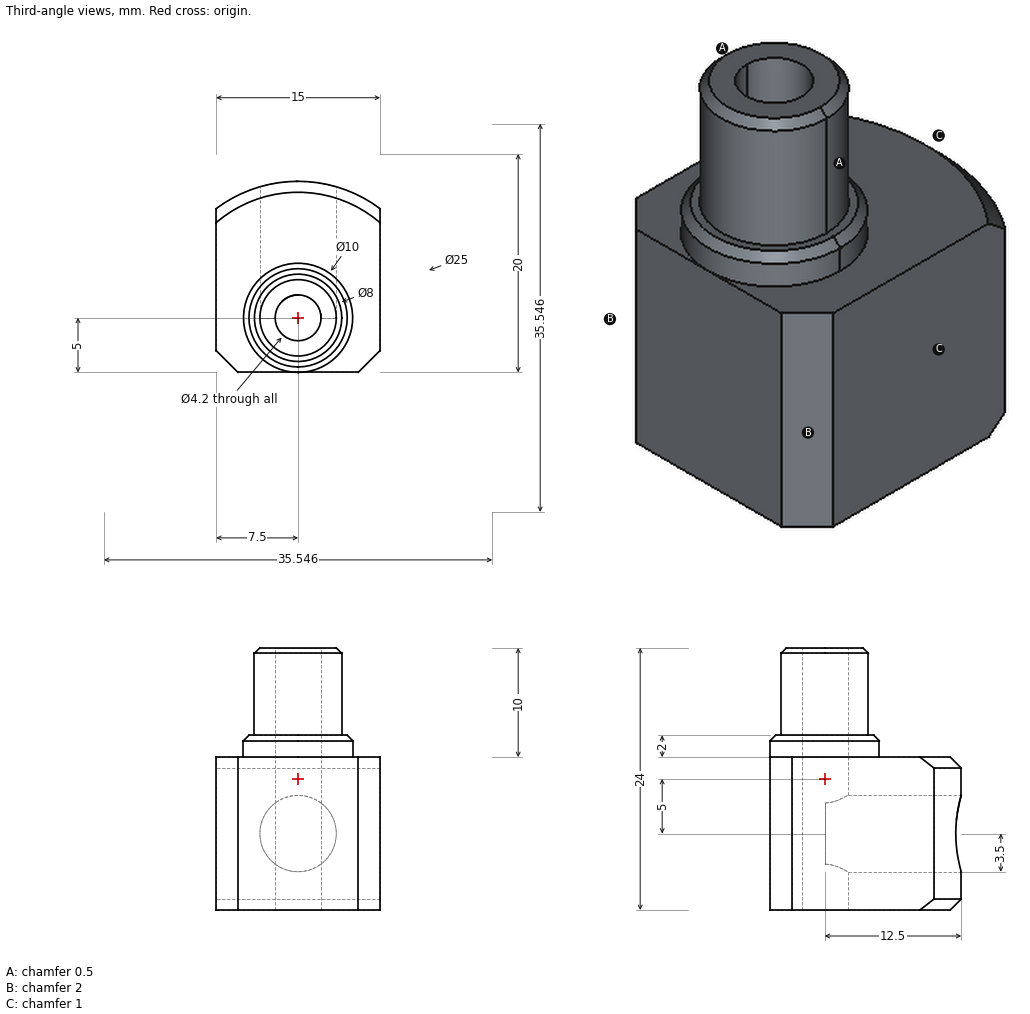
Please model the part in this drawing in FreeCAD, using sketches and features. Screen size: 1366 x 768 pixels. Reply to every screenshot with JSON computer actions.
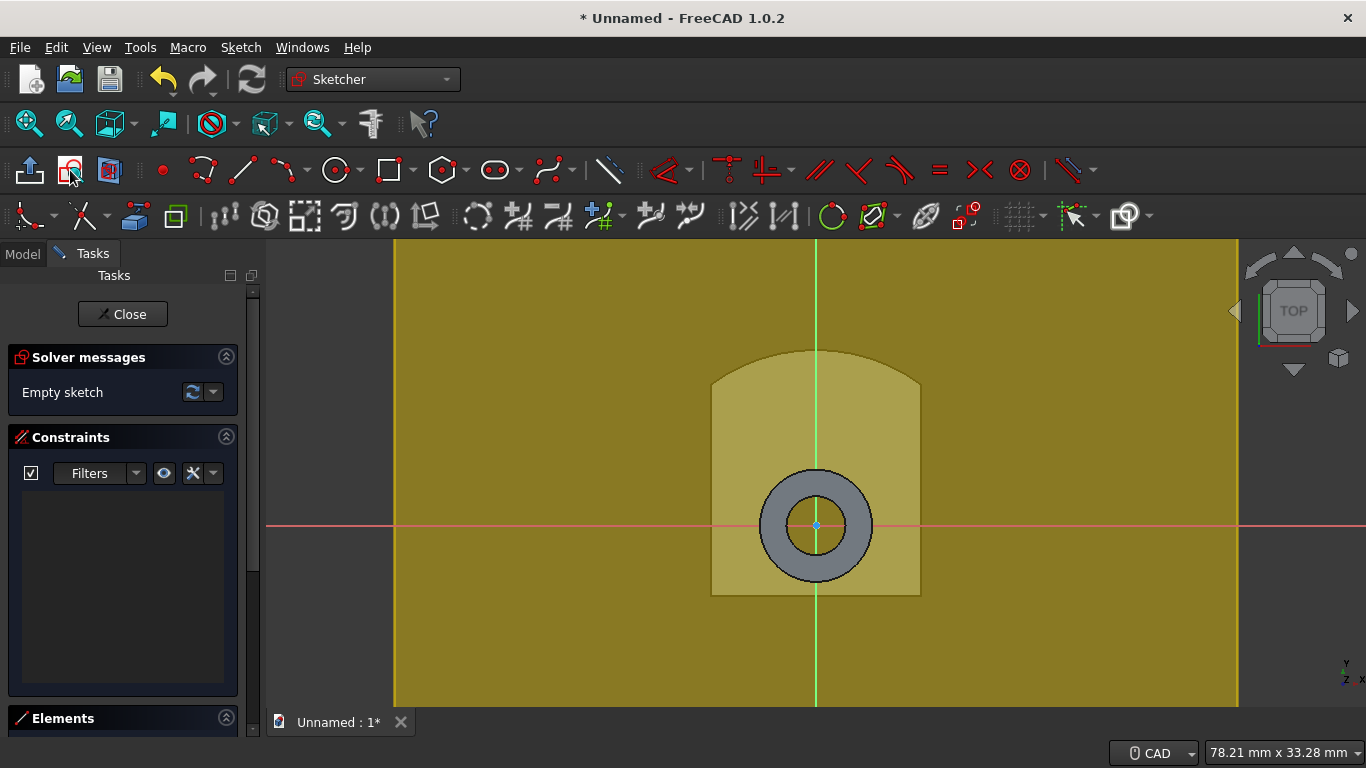
{"action": "left_click", "coordinate": [110, 170]}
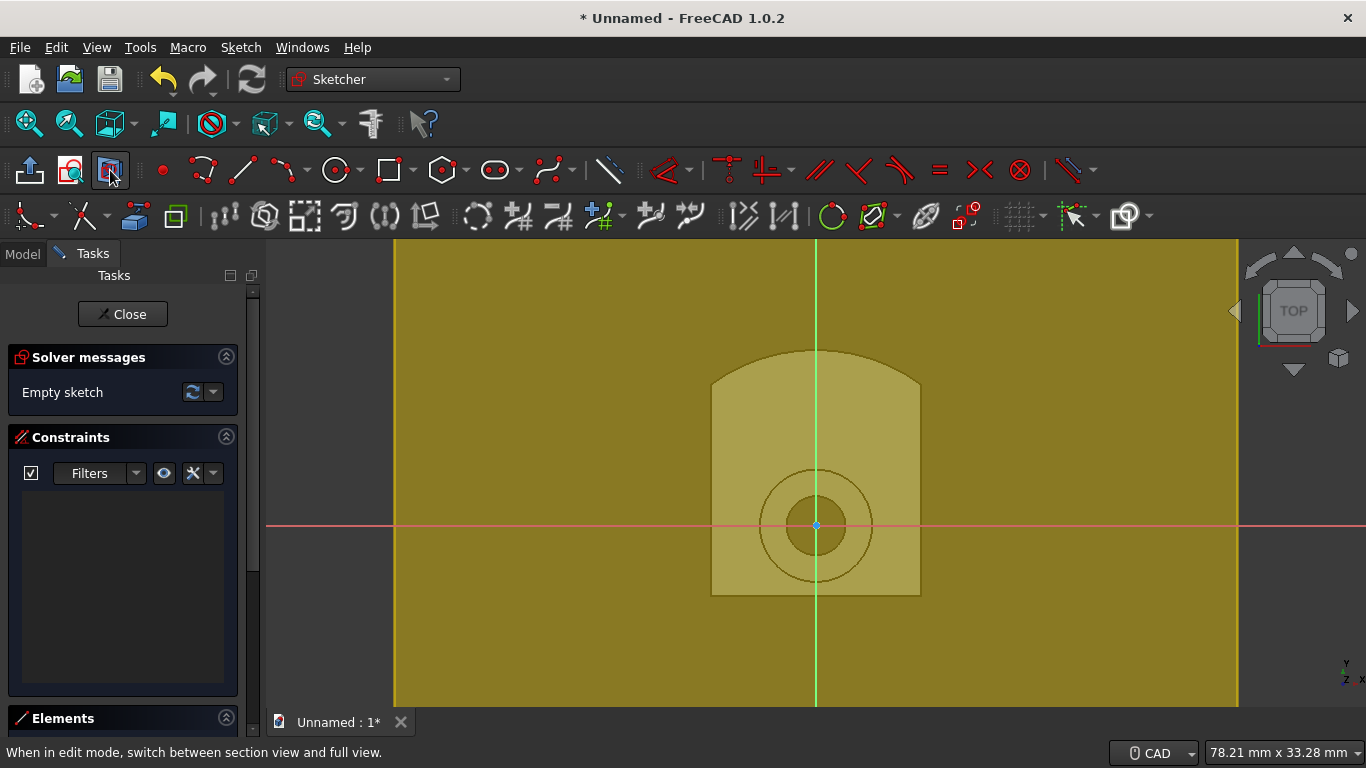
{"action": "scroll", "coordinate": [872, 569], "scroll_direction": "up", "scroll_amount": 4}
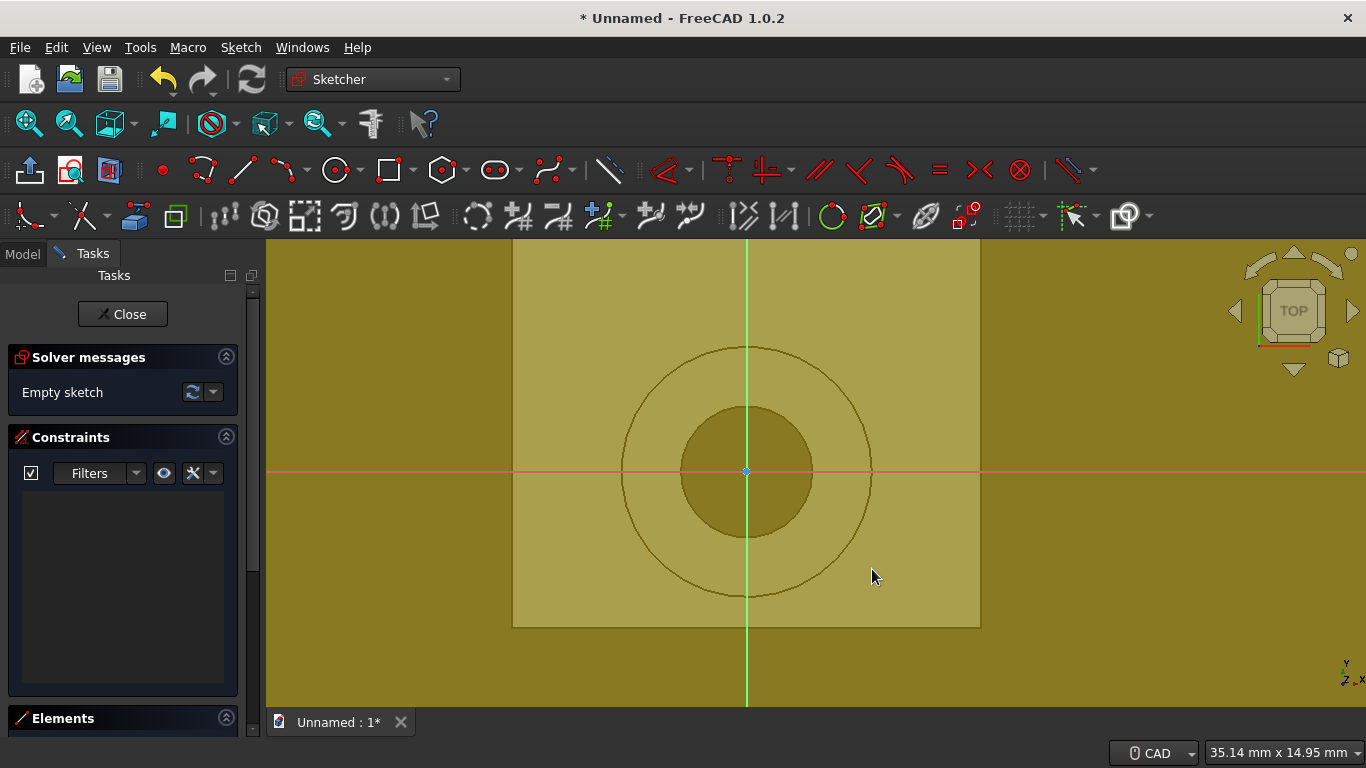
{"action": "left_click", "coordinate": [336, 170]}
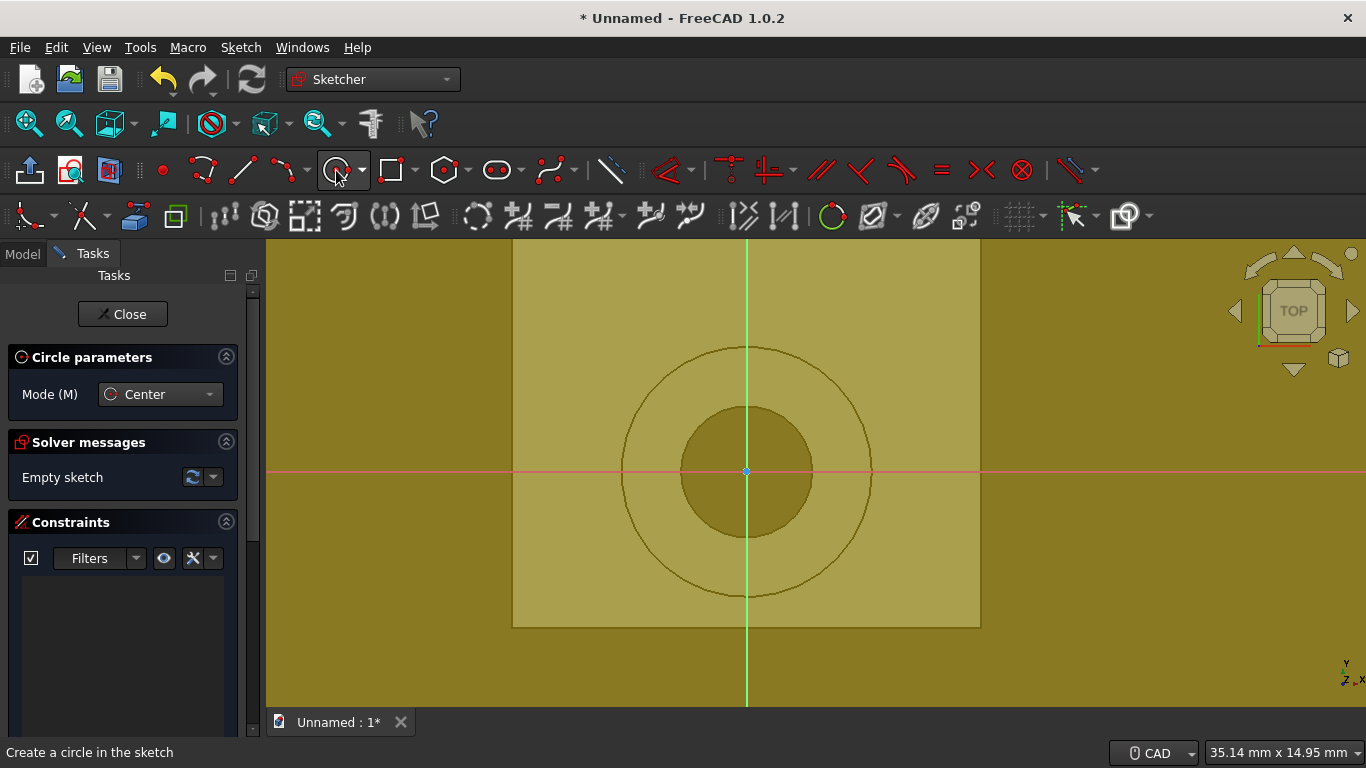
{"action": "left_click", "coordinate": [747, 472]}
{"action": "mouse_move", "coordinate": [857, 361]}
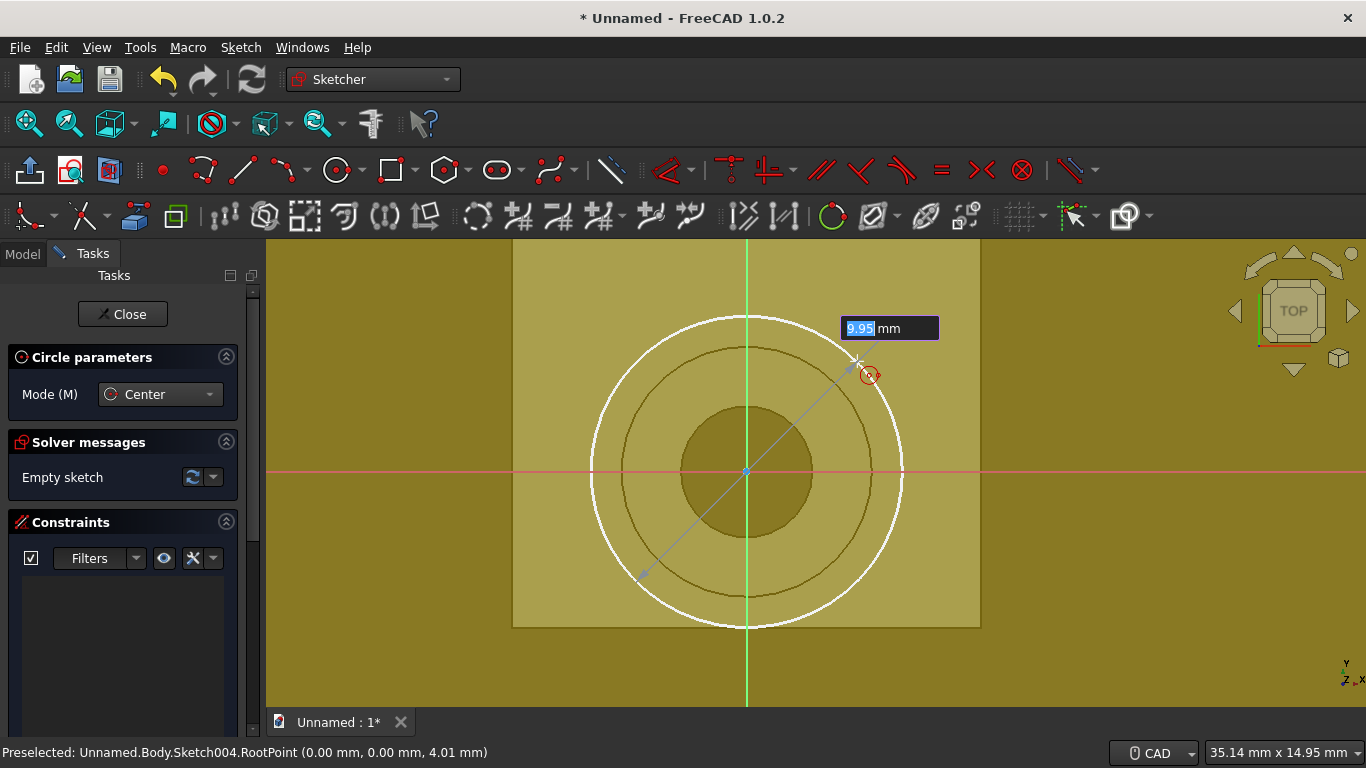
{"action": "type", "text": "10"}
{"action": "key", "text": "Return"}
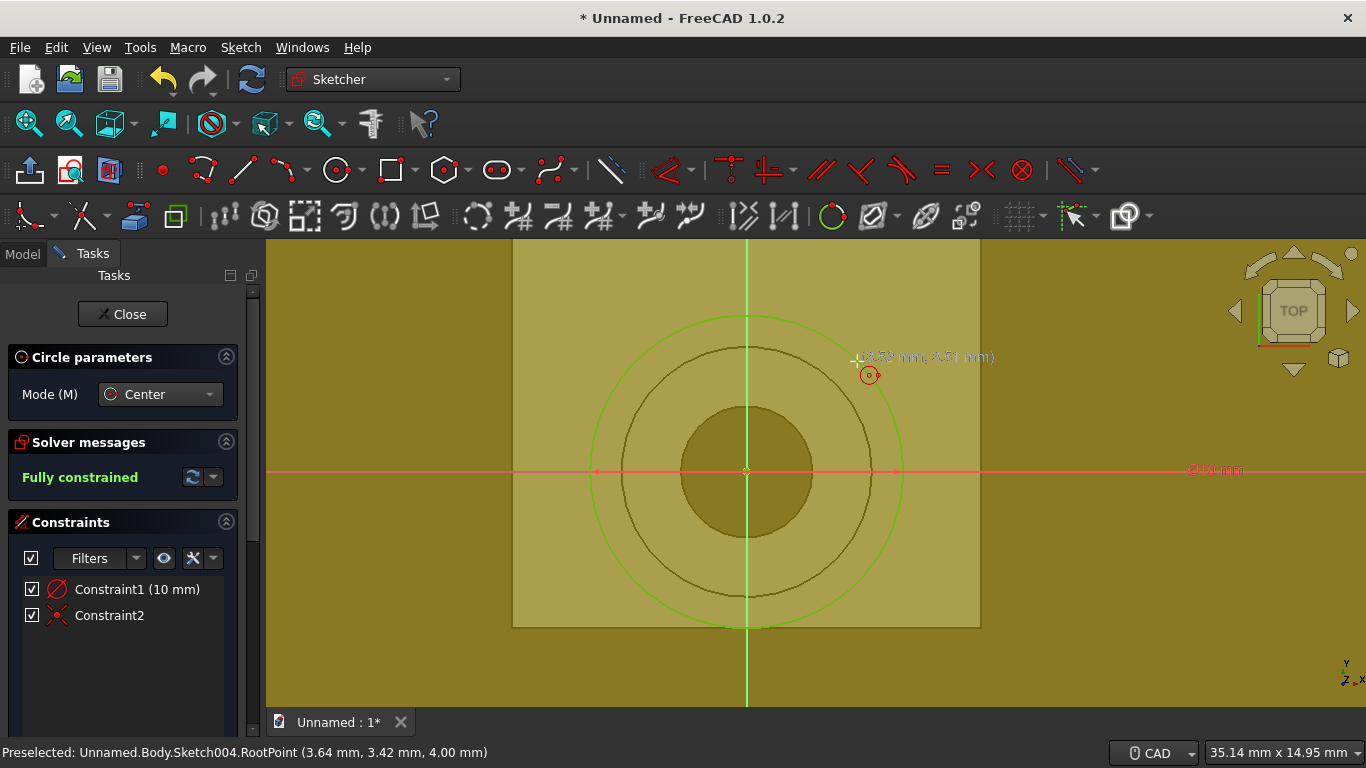
{"action": "left_click", "coordinate": [747, 472]}
{"action": "mouse_move", "coordinate": [835, 383]}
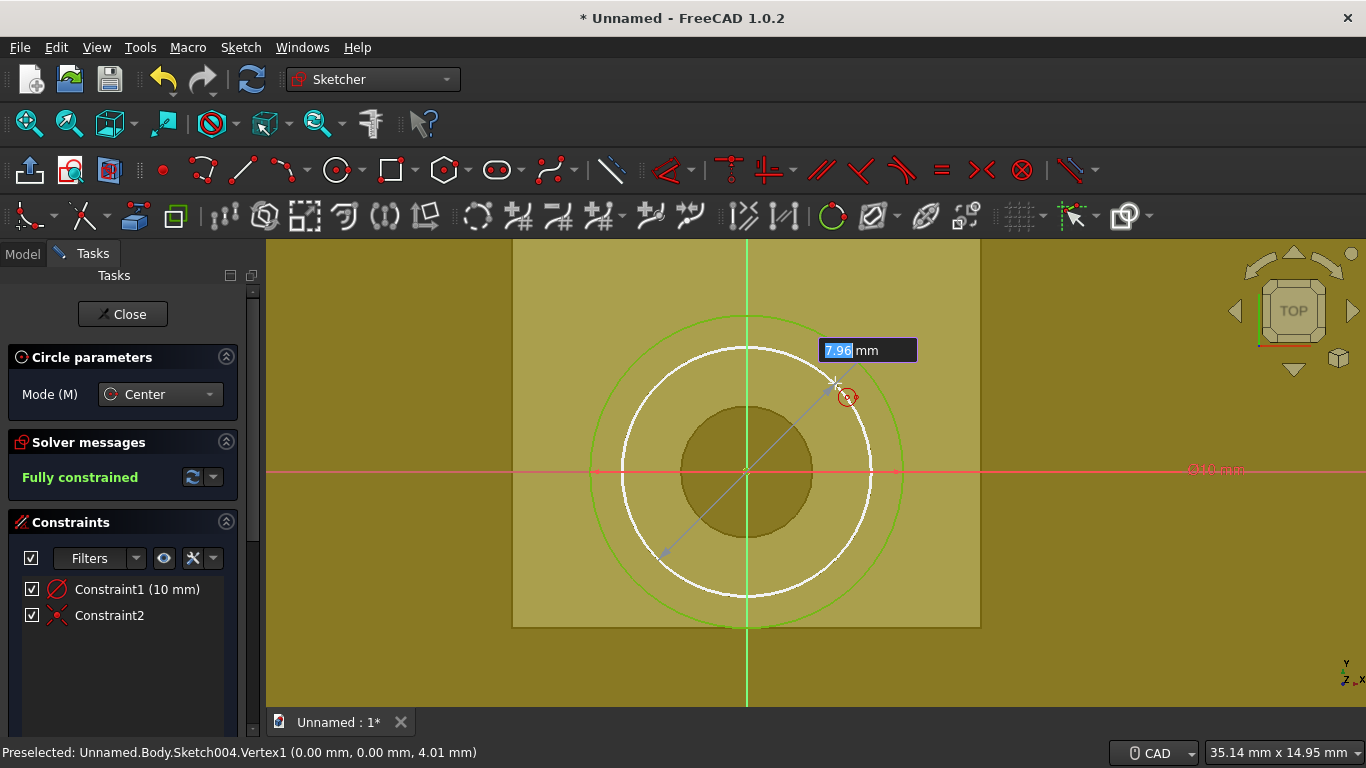
{"action": "type", "text": "8"}
{"action": "key", "text": "Return"}
{"action": "key", "text": "Escape"}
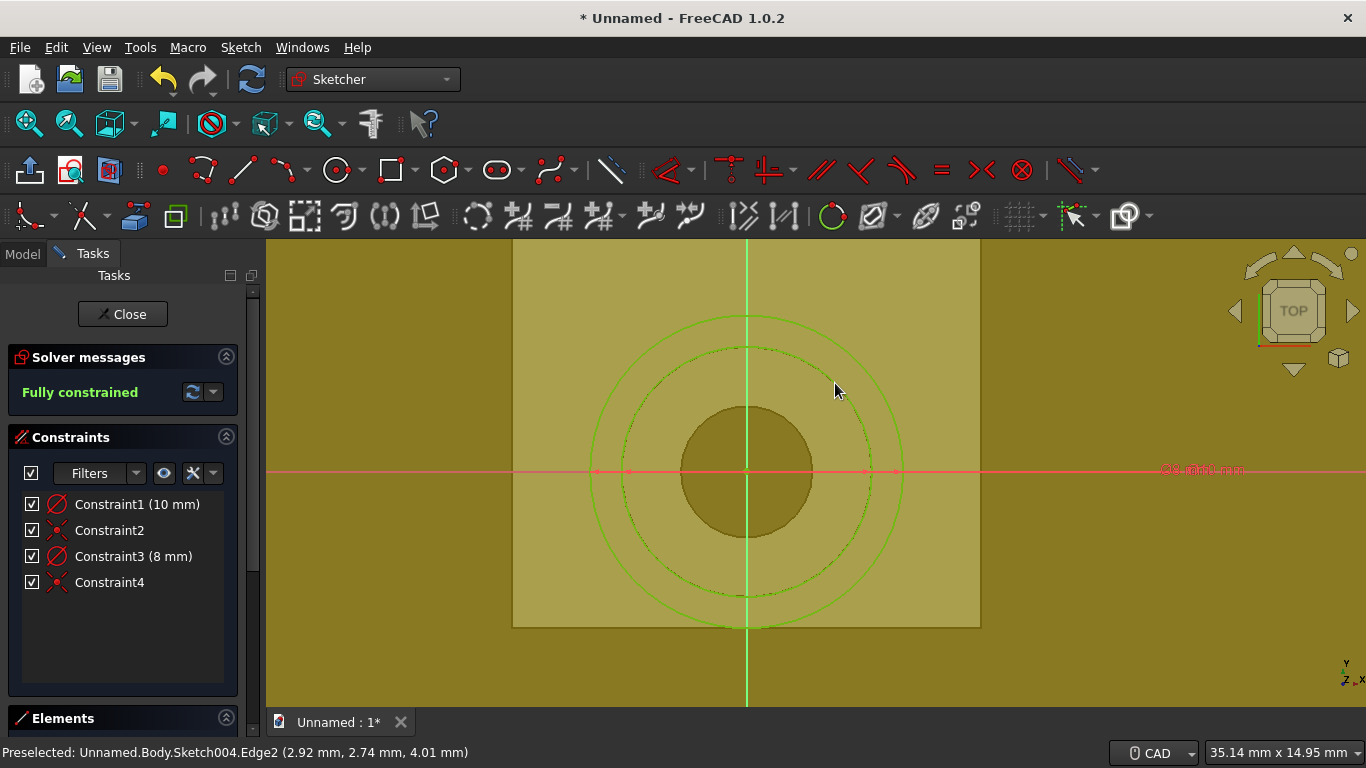
{"action": "left_click", "coordinate": [123, 314]}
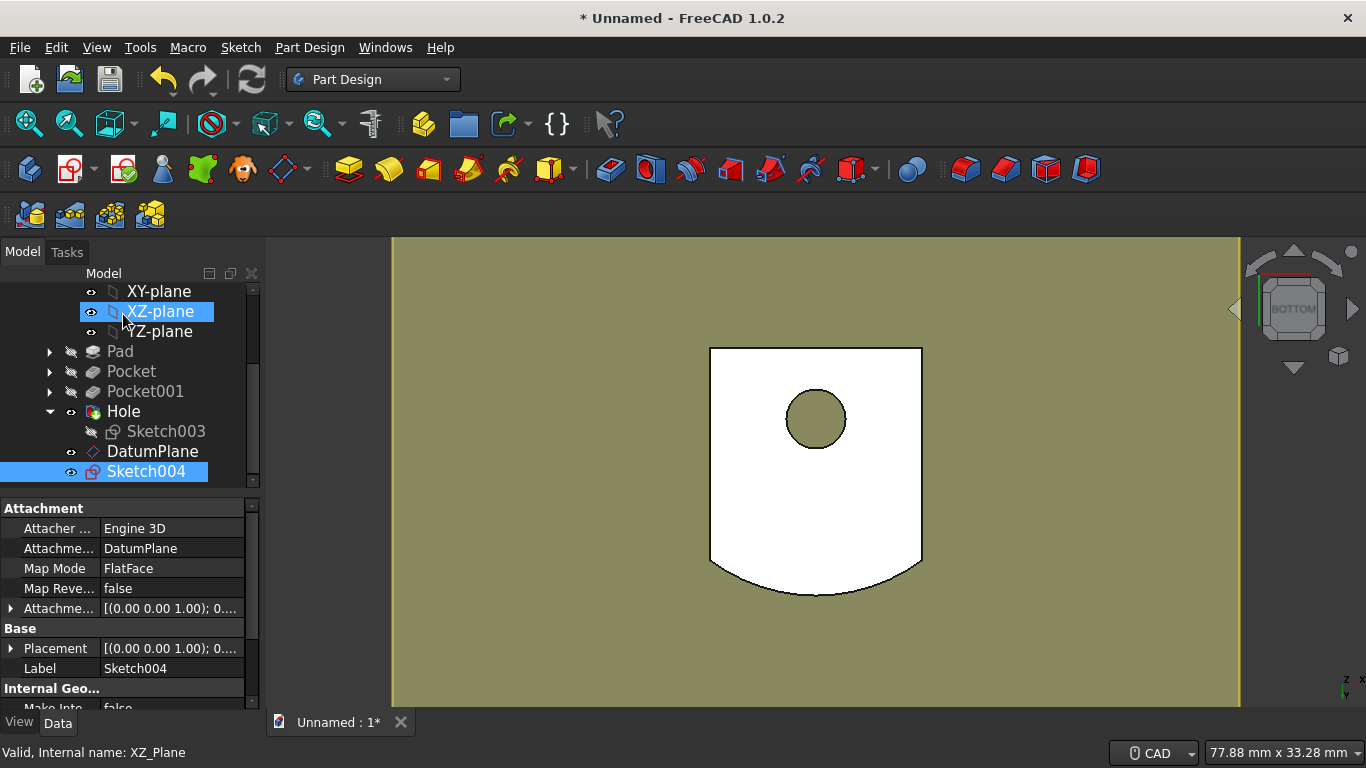
{"action": "left_click", "coordinate": [350, 170]}